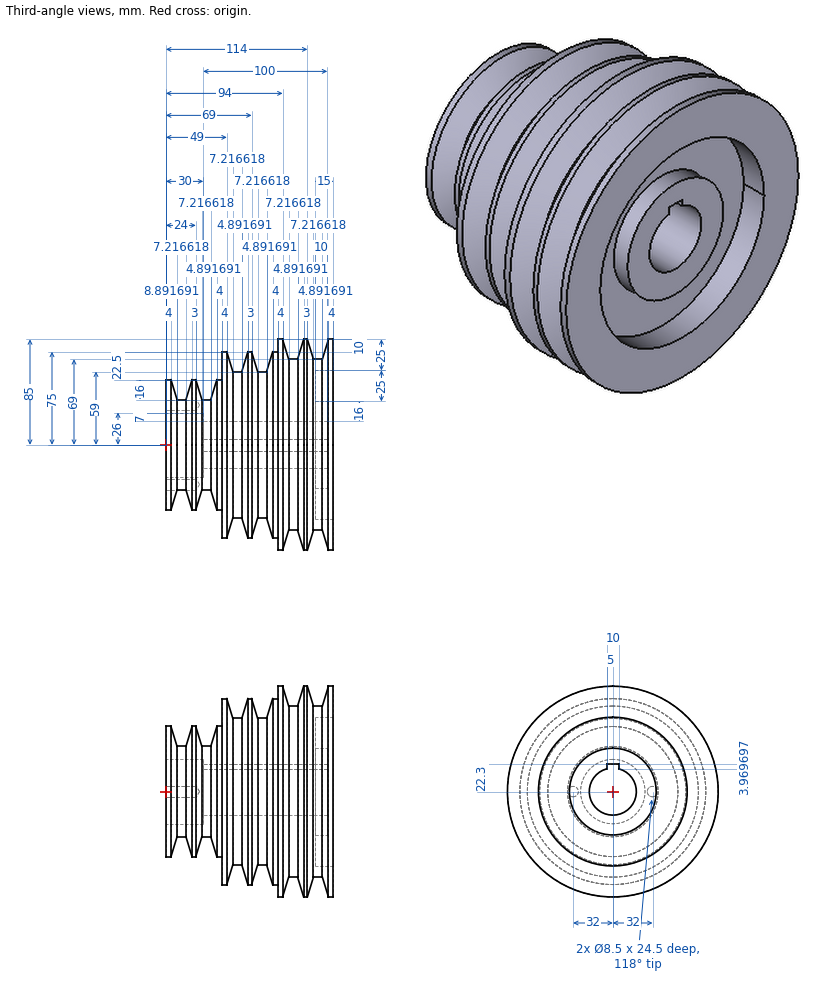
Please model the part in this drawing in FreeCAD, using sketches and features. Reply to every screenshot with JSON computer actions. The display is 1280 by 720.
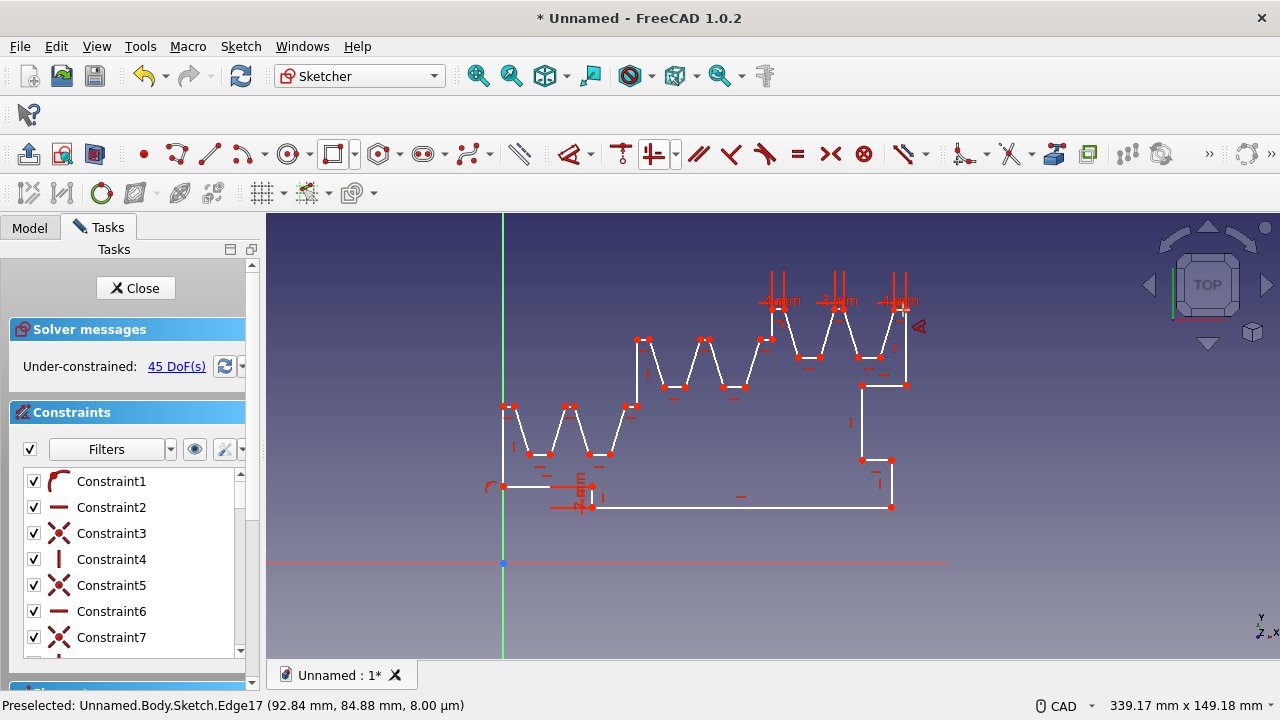
{"action": "scroll", "coordinate": [769, 340], "scroll_direction": "up", "scroll_amount": 7}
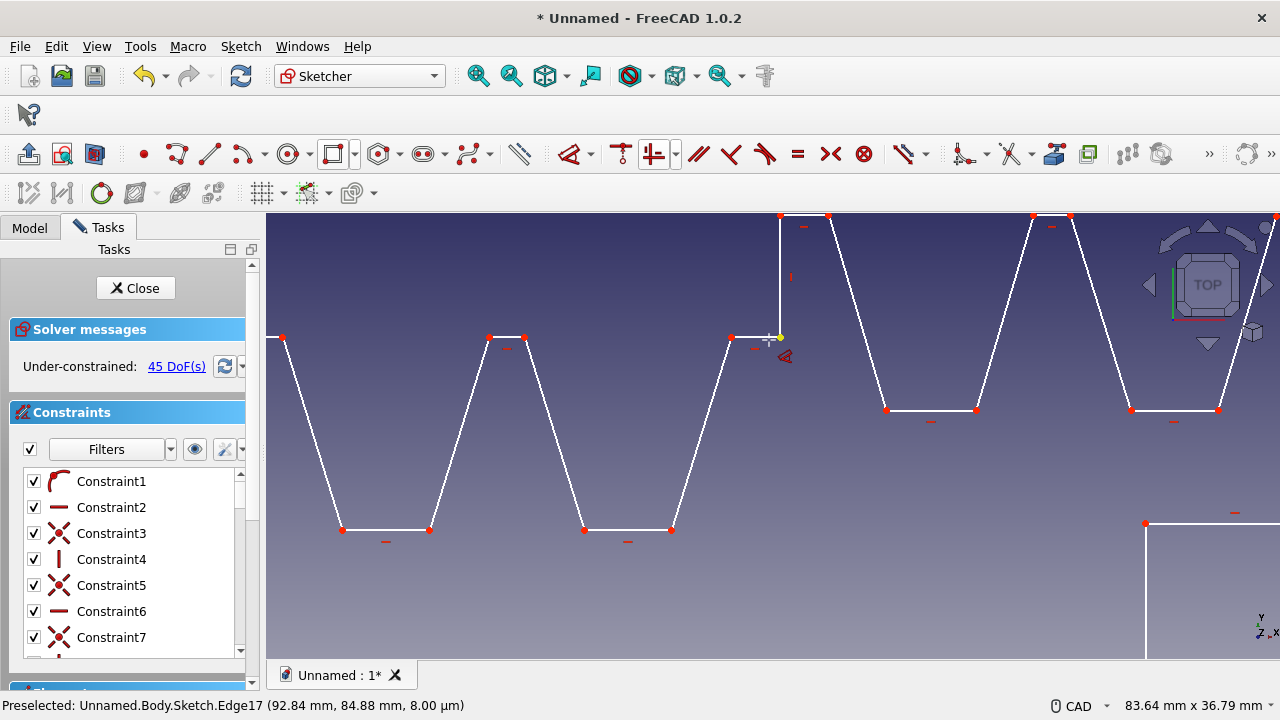
{"action": "left_click", "coordinate": [766, 337]}
{"action": "left_click", "coordinate": [756, 303]}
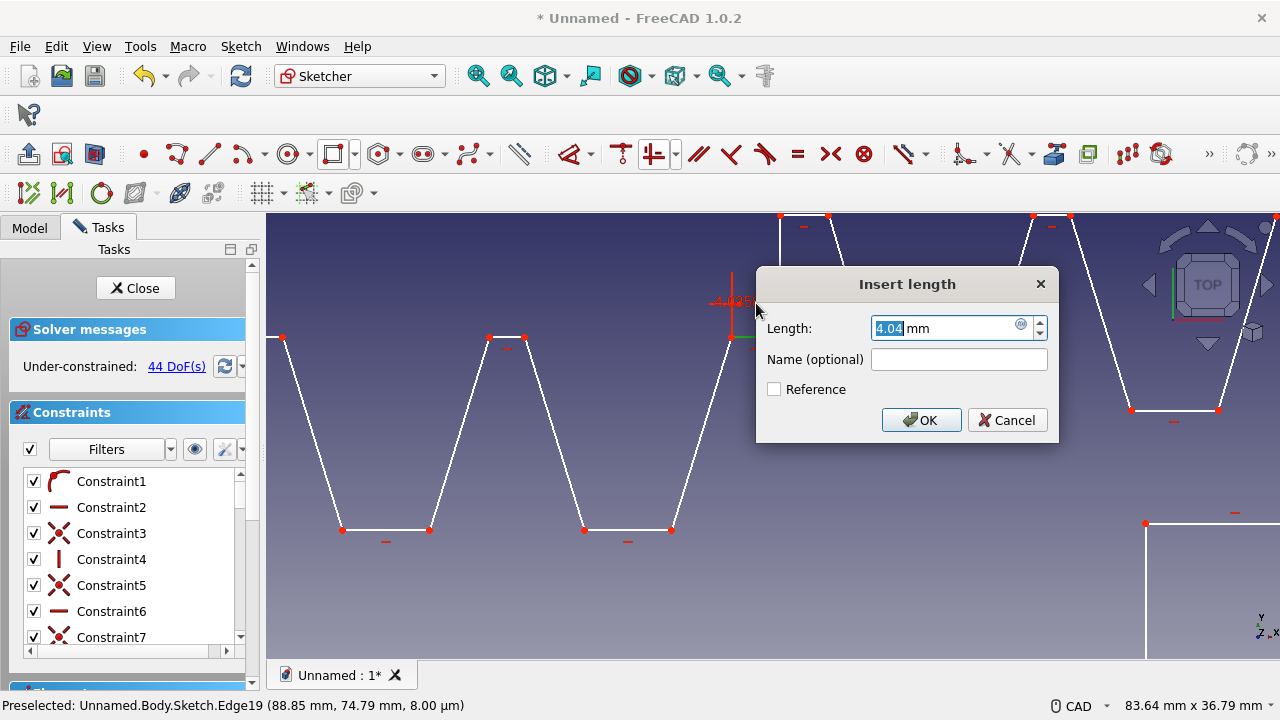
{"action": "type", "text": "4"}
{"action": "key", "text": "Return"}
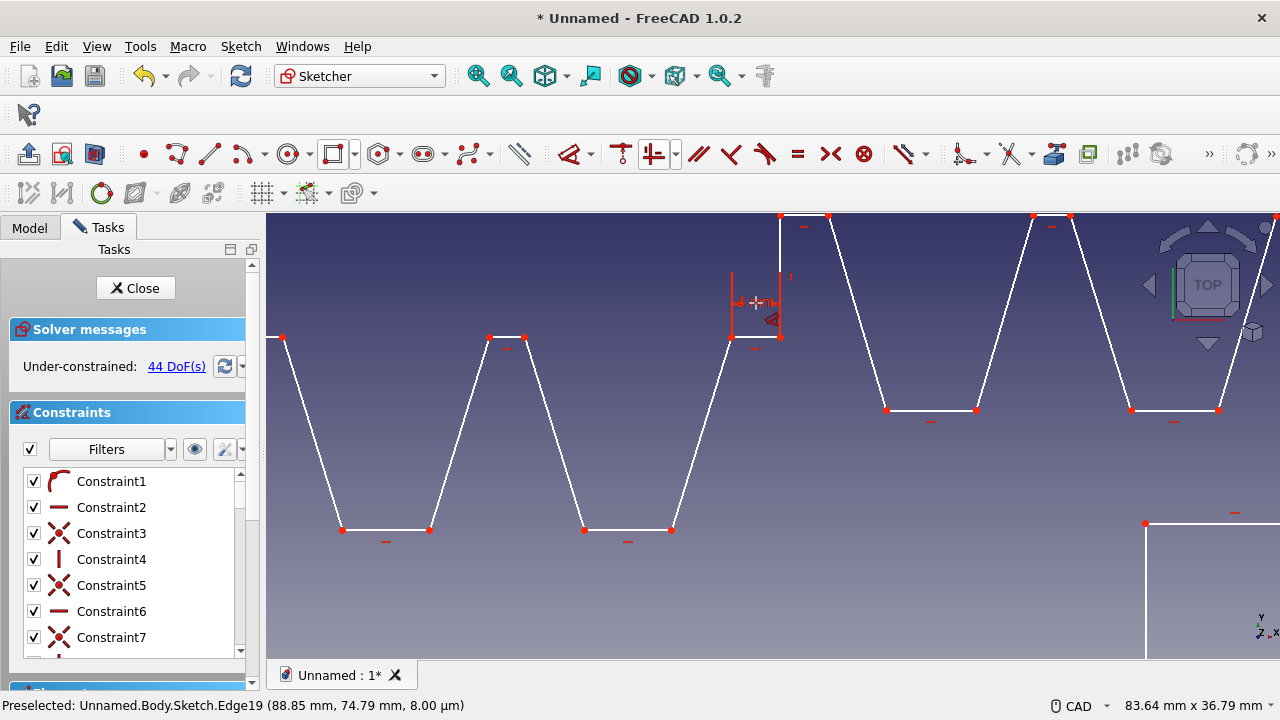
{"action": "scroll", "coordinate": [514, 337], "scroll_direction": "up", "scroll_amount": 2}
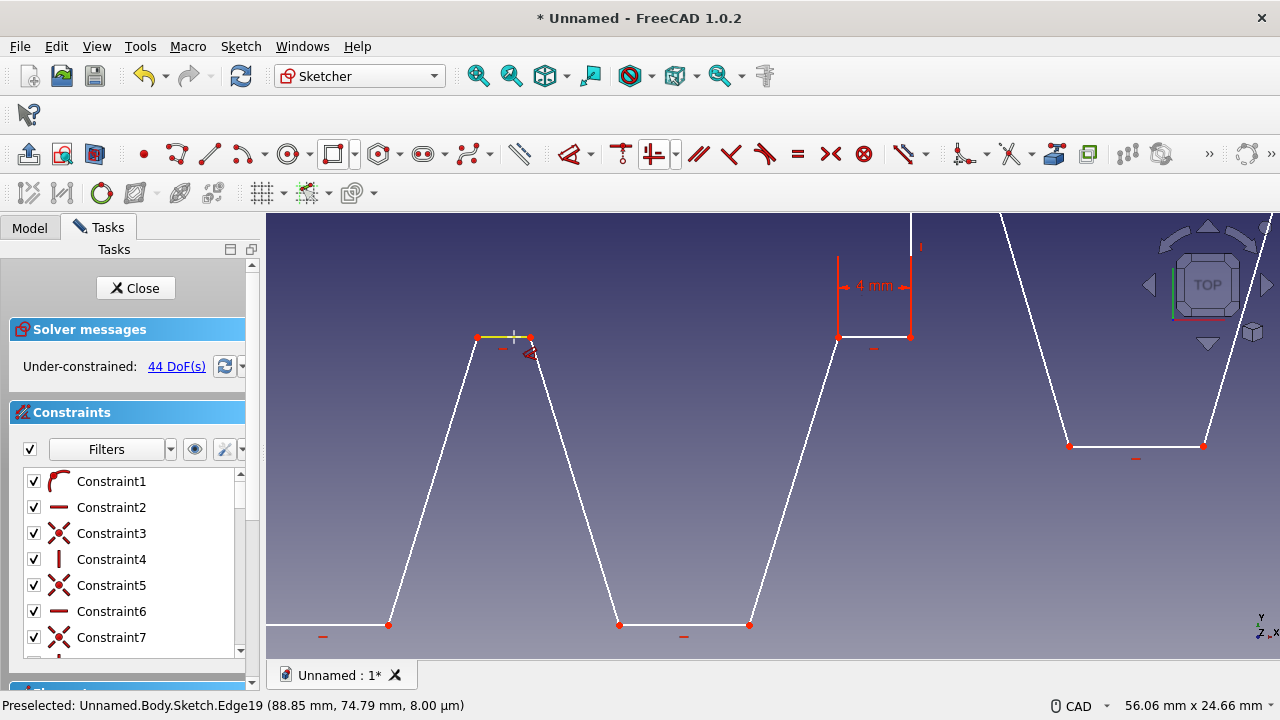
{"action": "left_click", "coordinate": [514, 337]}
{"action": "left_click", "coordinate": [504, 303]}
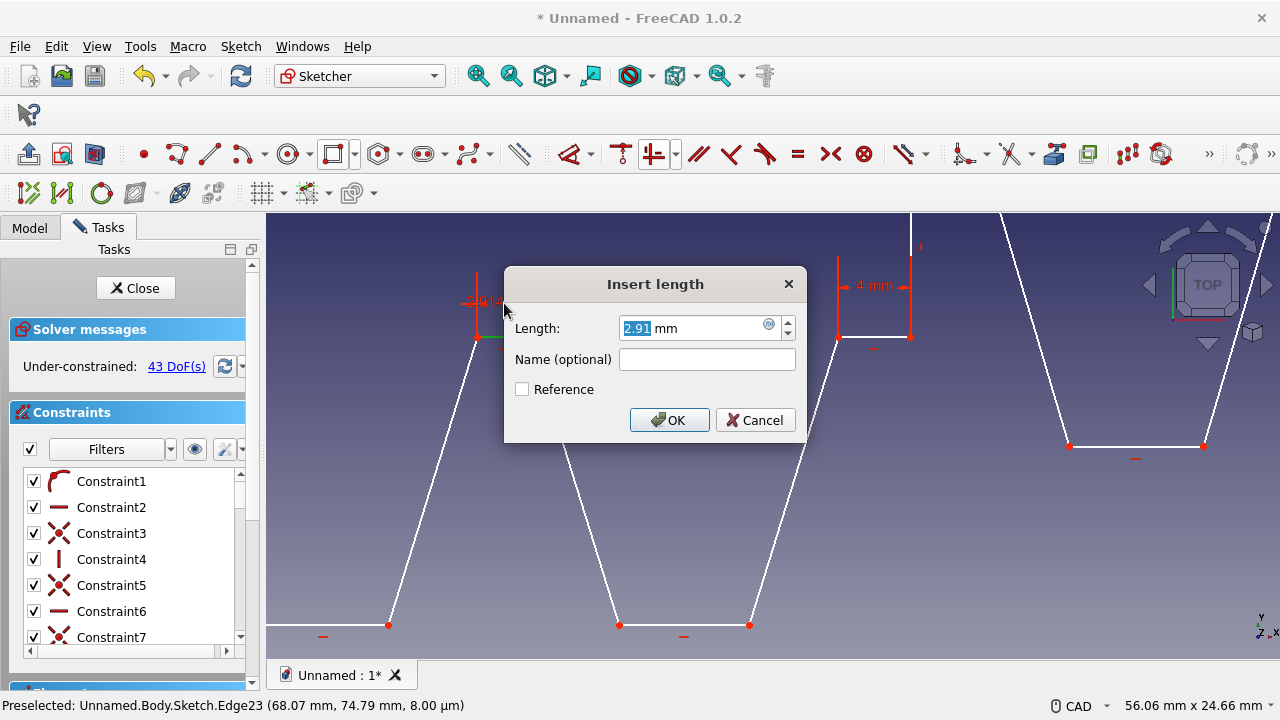
{"action": "type", "text": "3"}
{"action": "key", "text": "Return"}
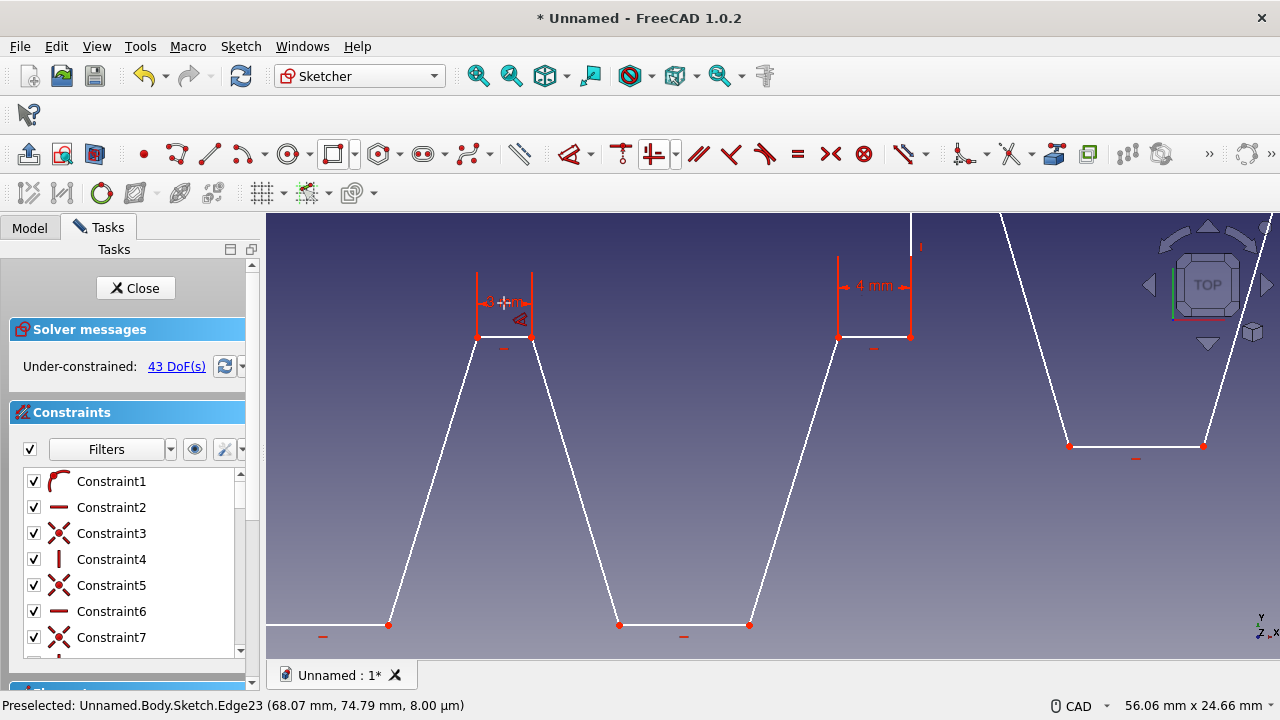
{"action": "scroll", "coordinate": [744, 340], "scroll_direction": "down", "scroll_amount": 9}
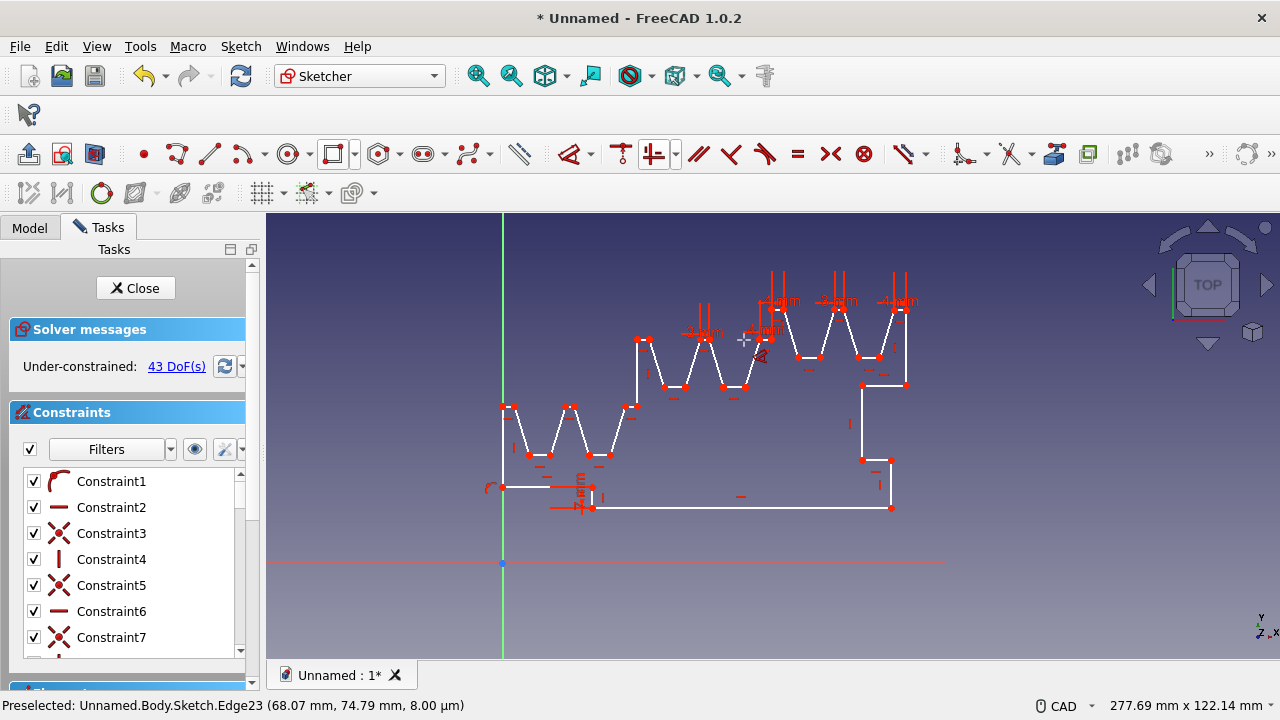
{"action": "scroll", "coordinate": [646, 340], "scroll_direction": "up", "scroll_amount": 7}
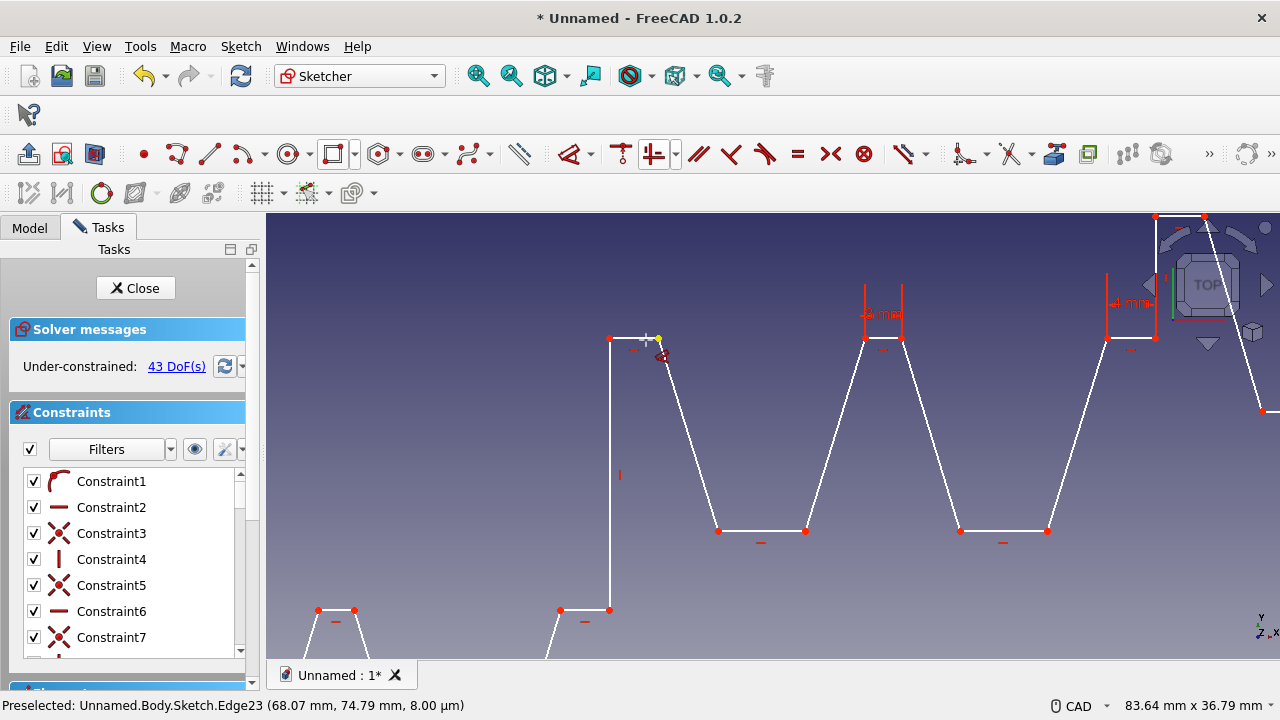
{"action": "left_click", "coordinate": [644, 338]}
{"action": "left_click", "coordinate": [634, 304]}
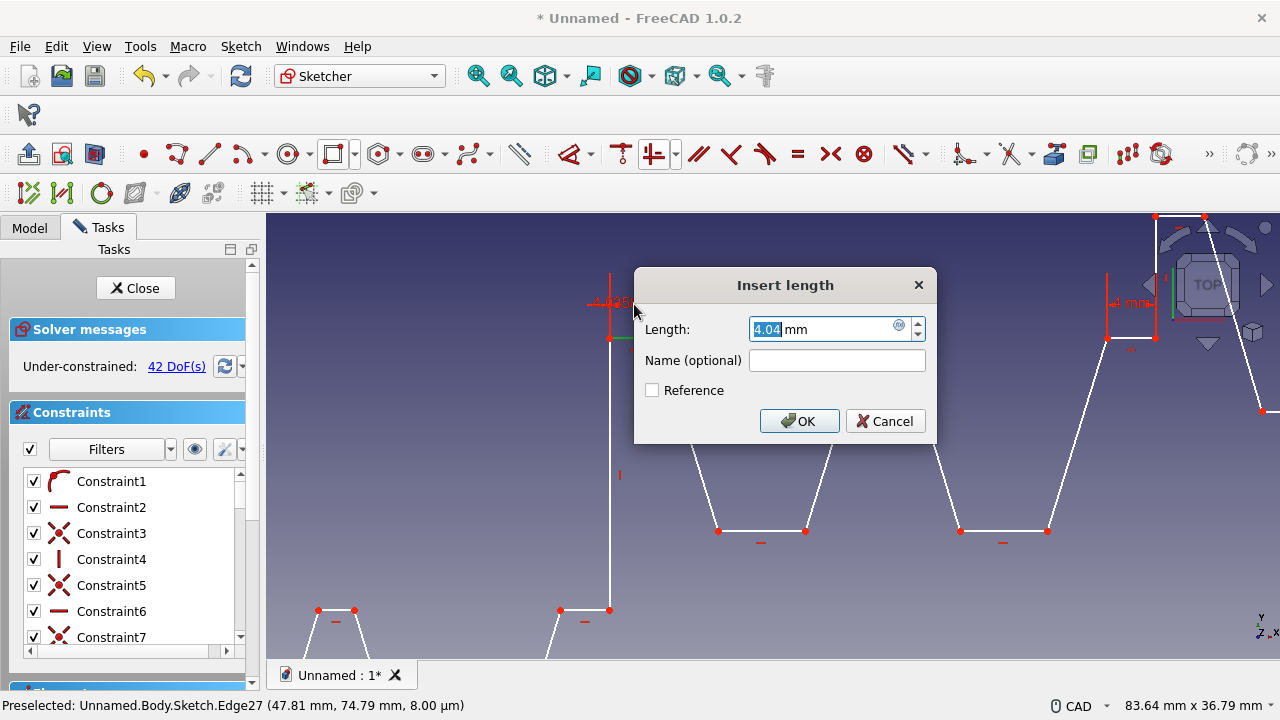
{"action": "type", "text": "4"}
{"action": "key", "text": "Return"}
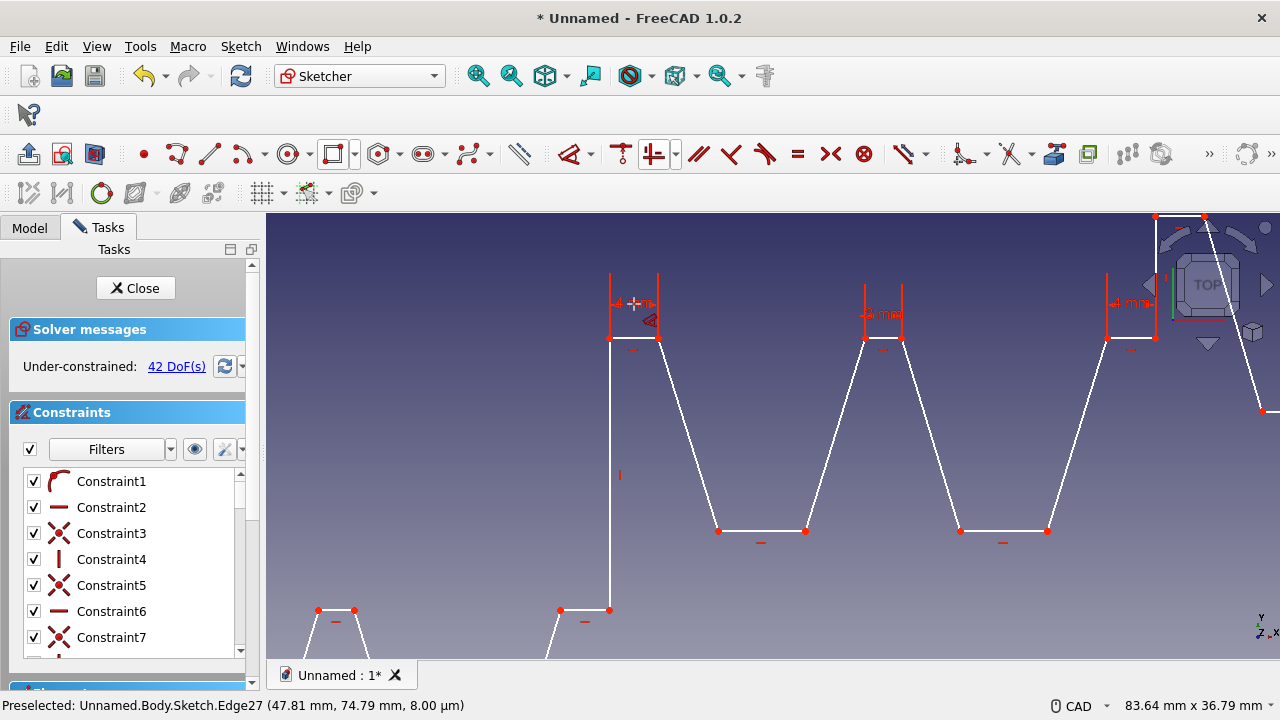
{"action": "left_click", "coordinate": [595, 610]}
{"action": "left_click", "coordinate": [585, 576]}